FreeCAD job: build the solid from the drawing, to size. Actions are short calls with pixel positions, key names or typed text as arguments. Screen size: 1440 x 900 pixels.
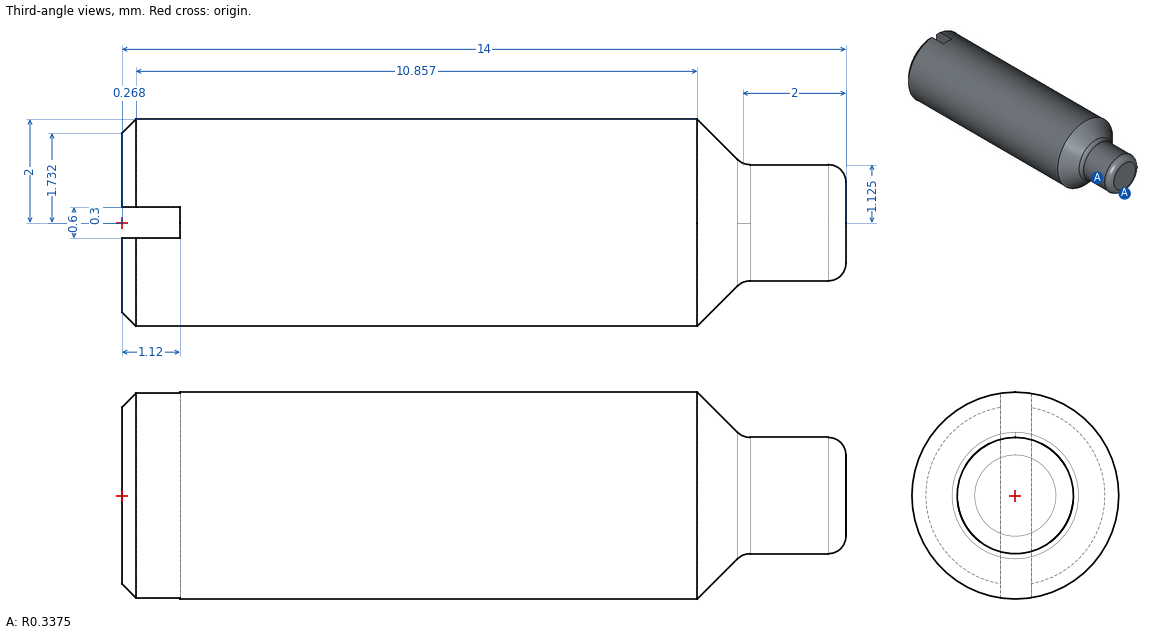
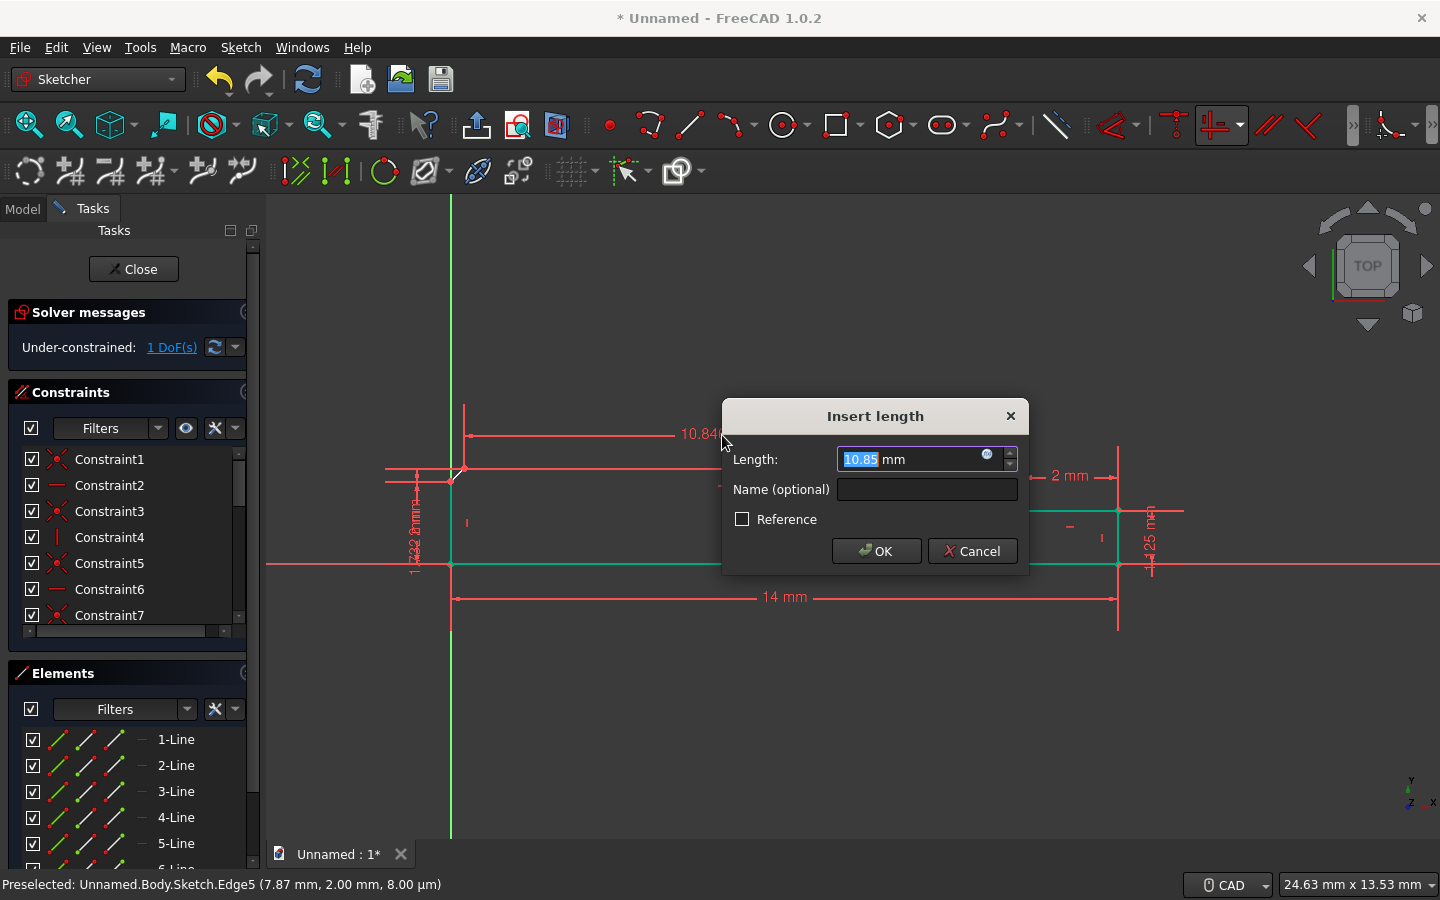
text(10.857)
key(Return)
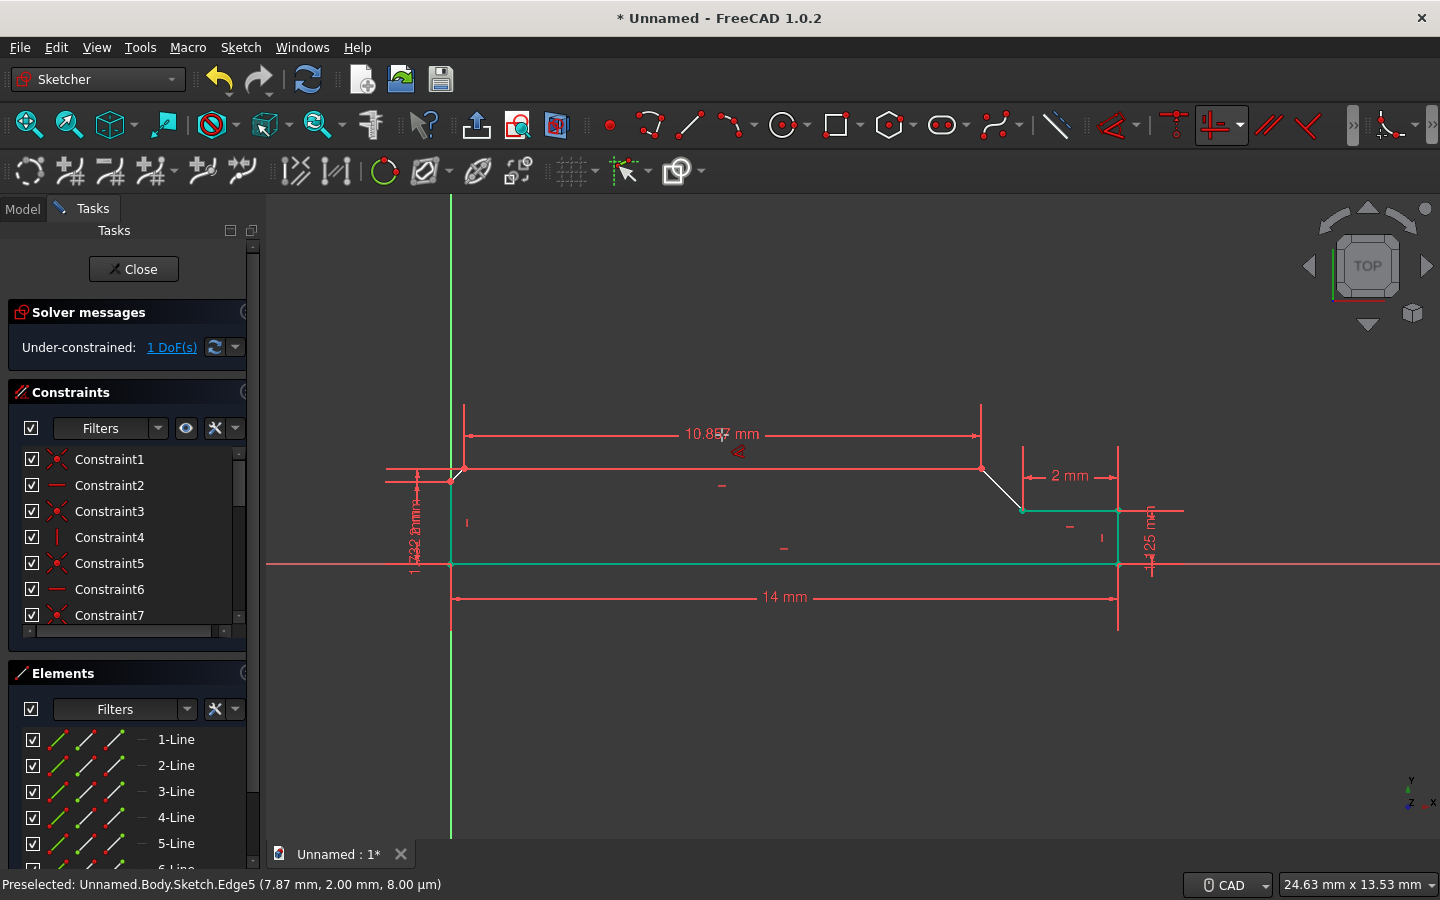
scroll(464, 469, up, 6)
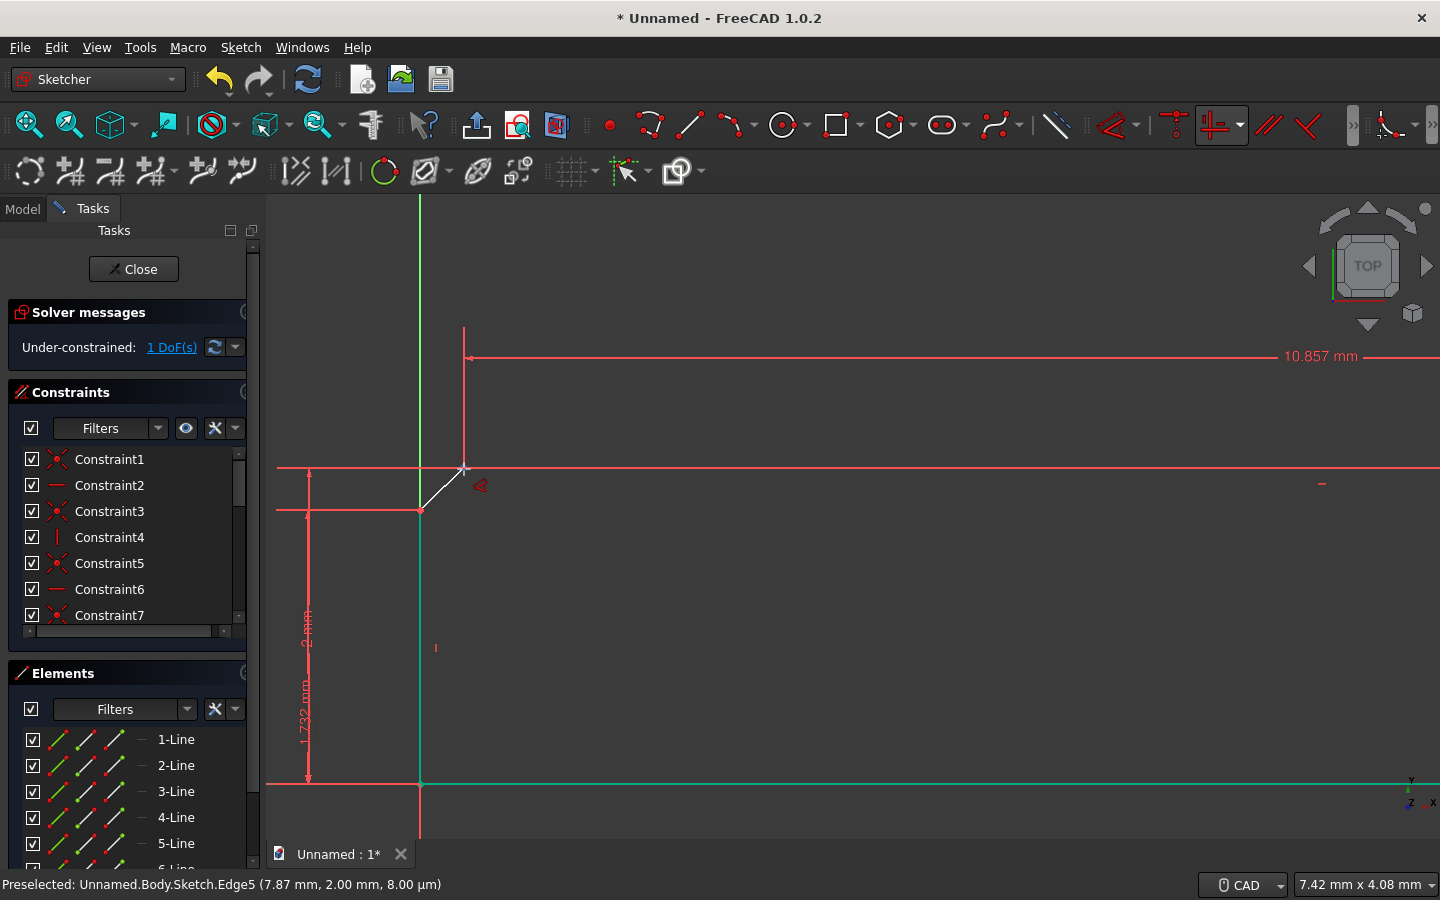
click(464, 468)
click(442, 434)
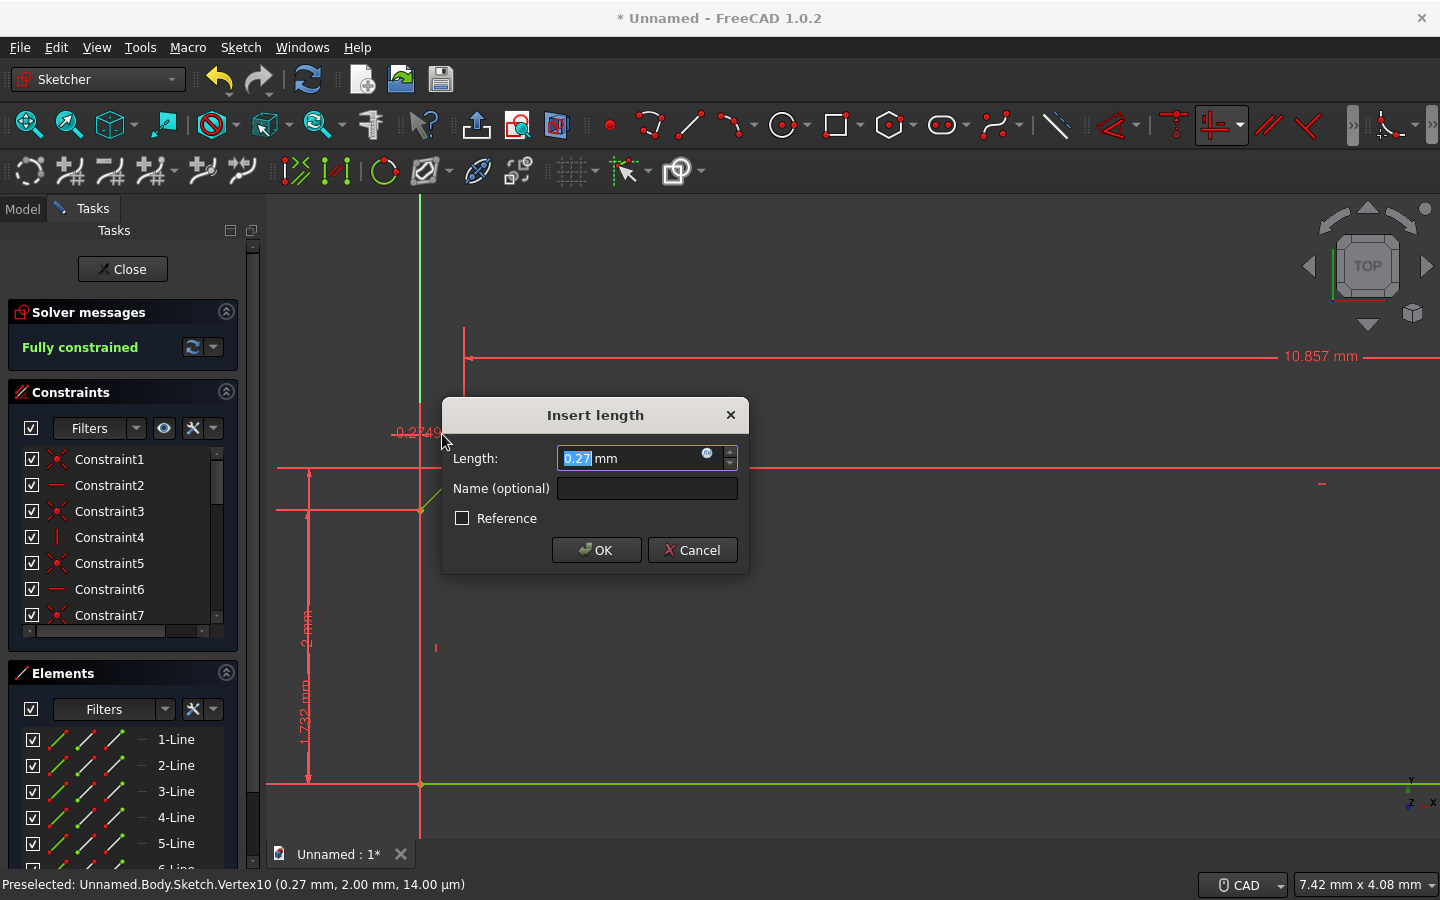
text(0.268)
key(Return)
key(Escape)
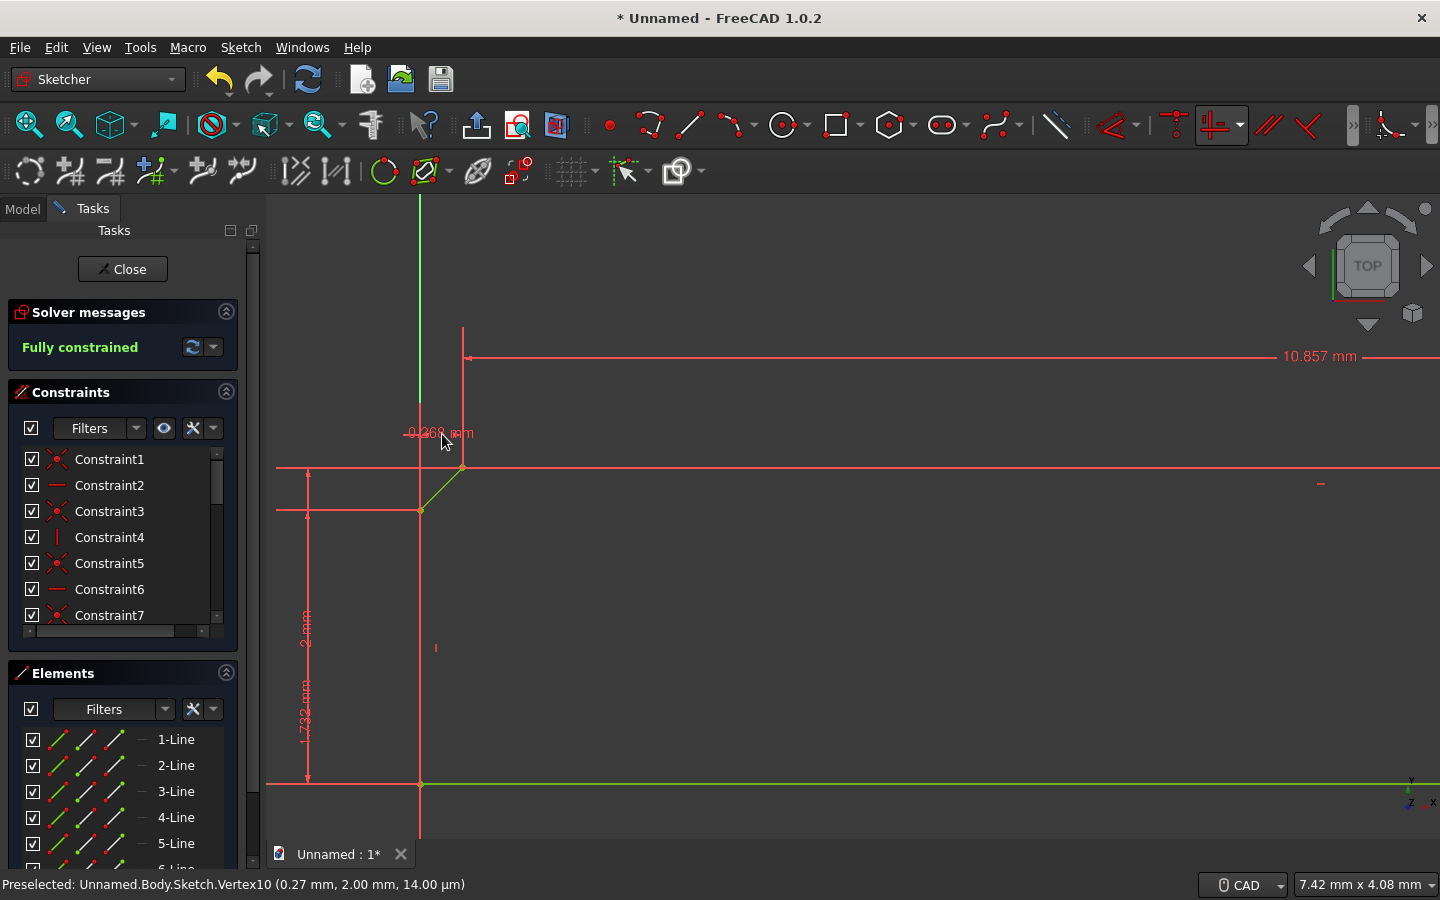
click(123, 269)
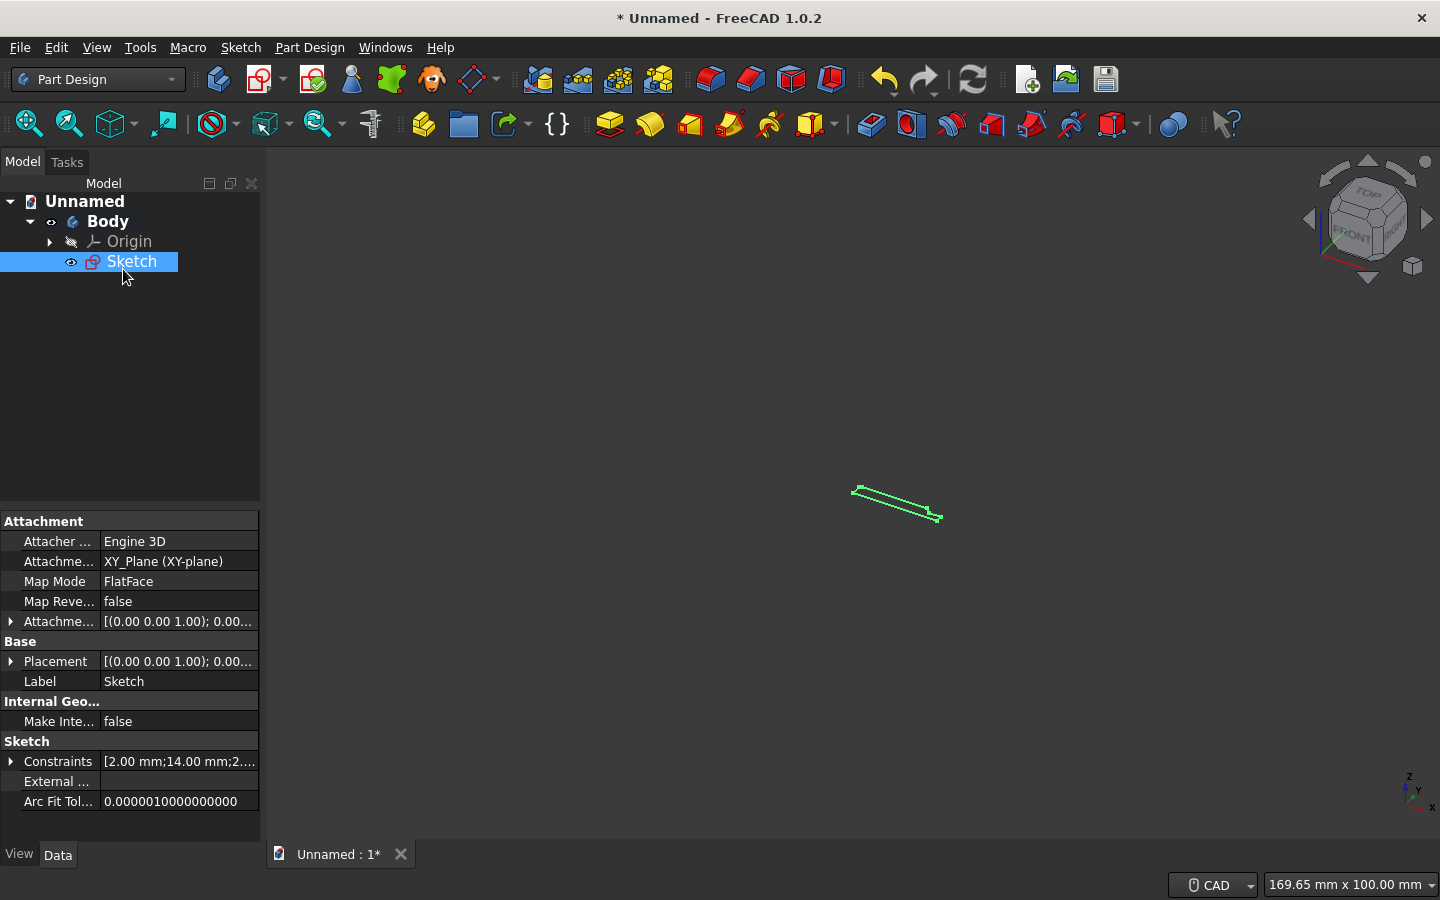
click(650, 124)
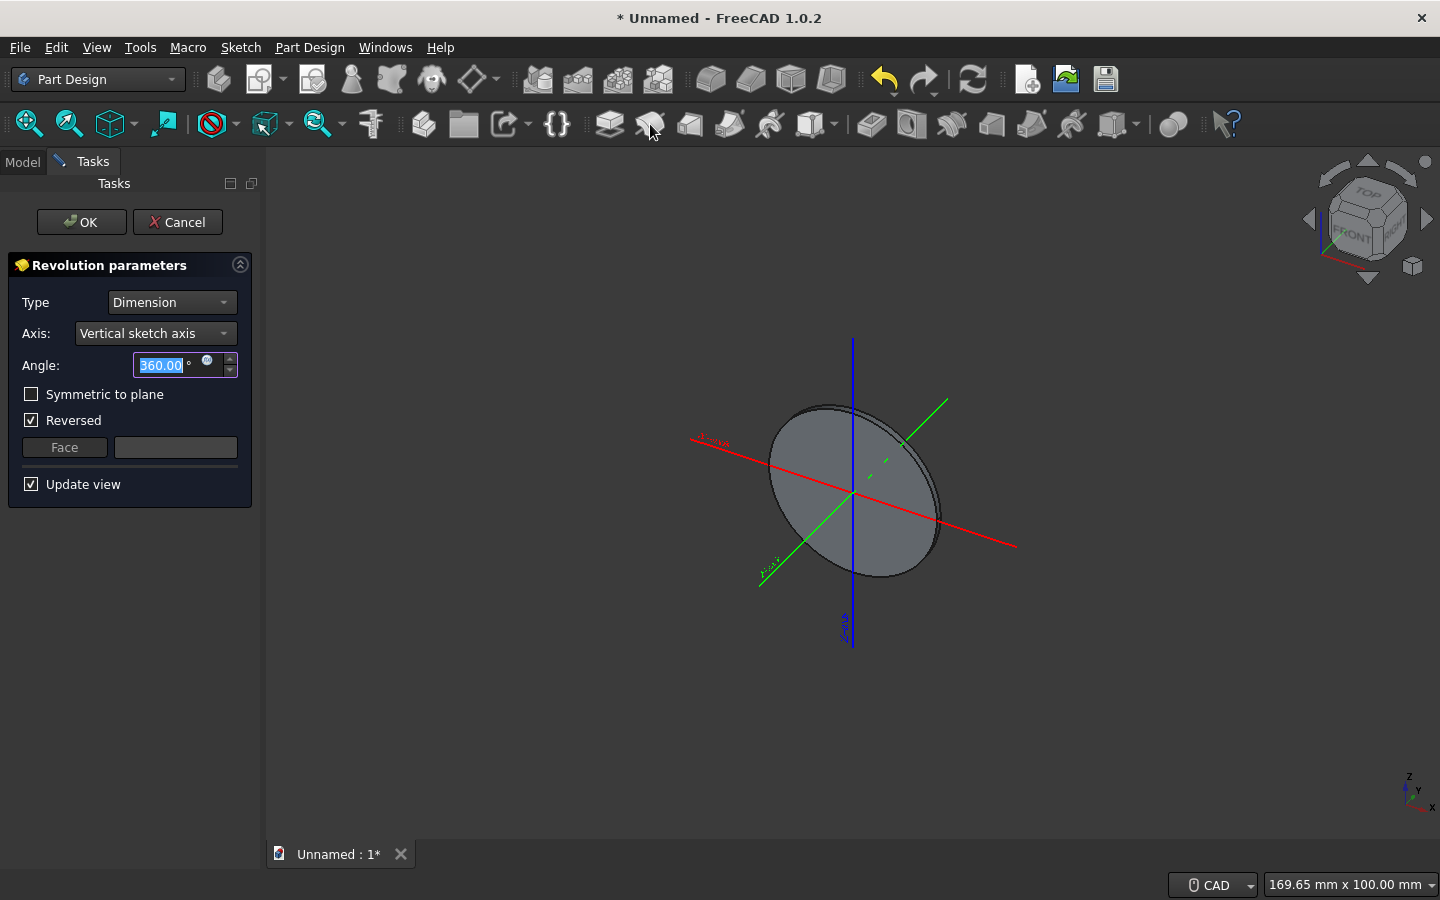
click(156, 334)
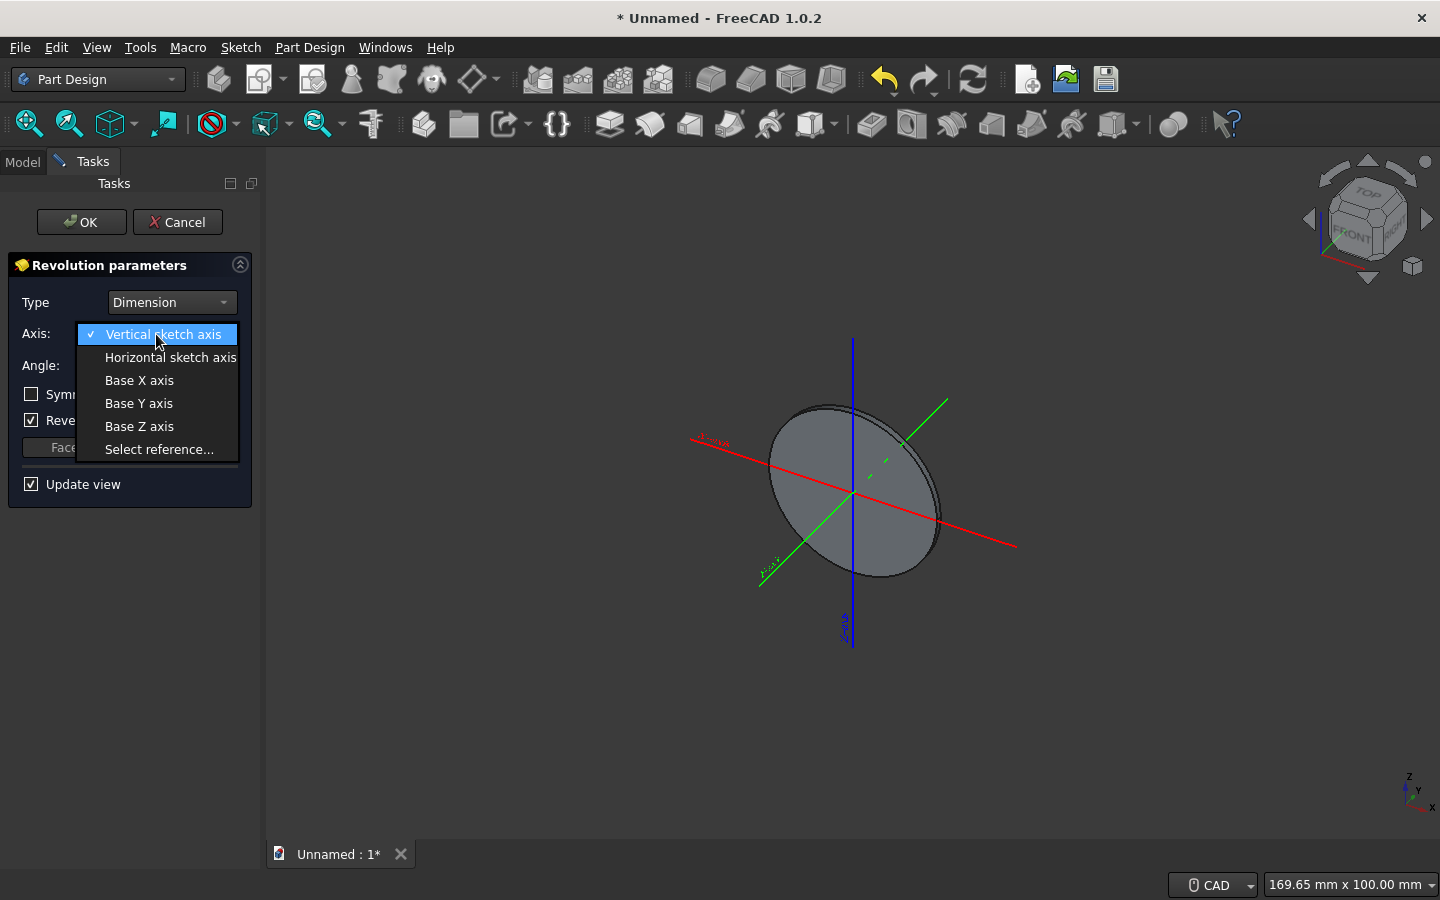
click(156, 358)